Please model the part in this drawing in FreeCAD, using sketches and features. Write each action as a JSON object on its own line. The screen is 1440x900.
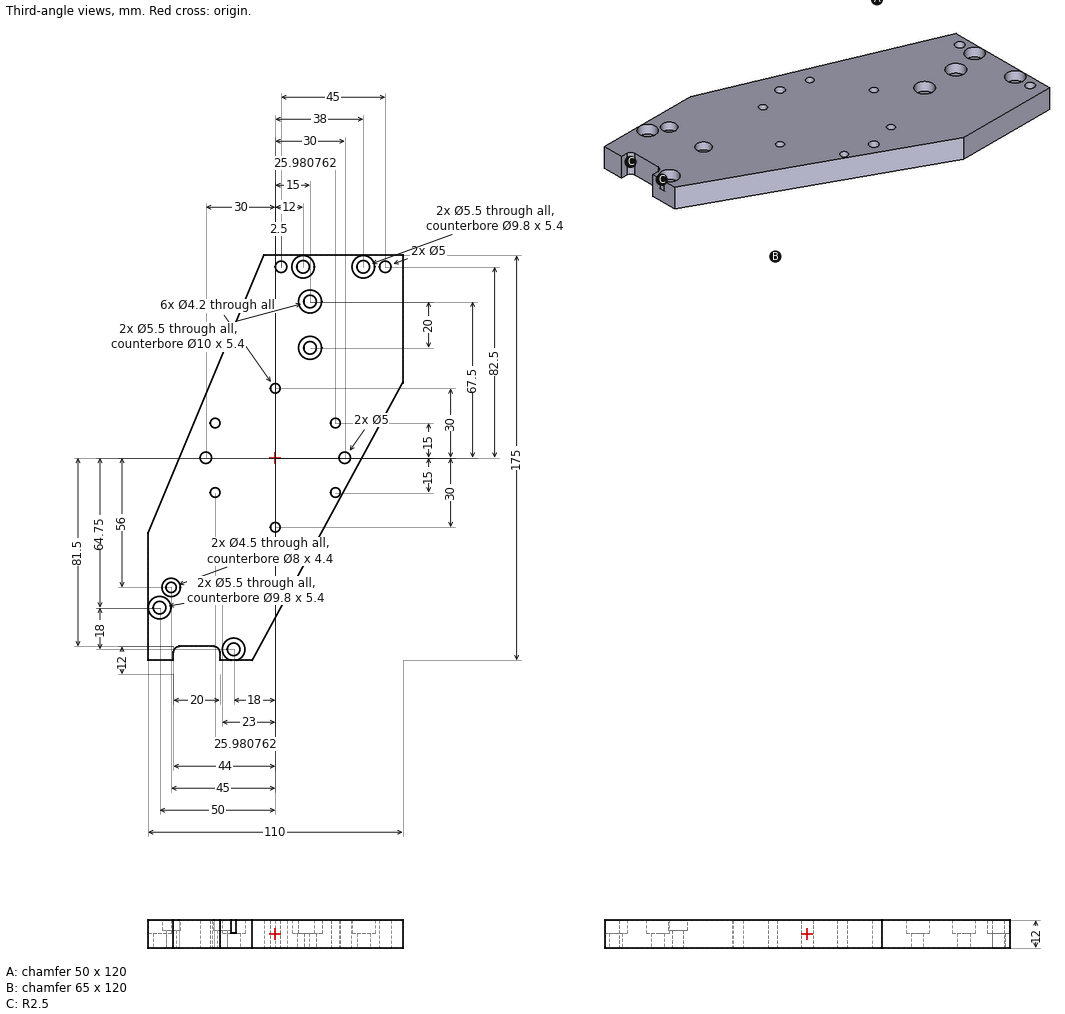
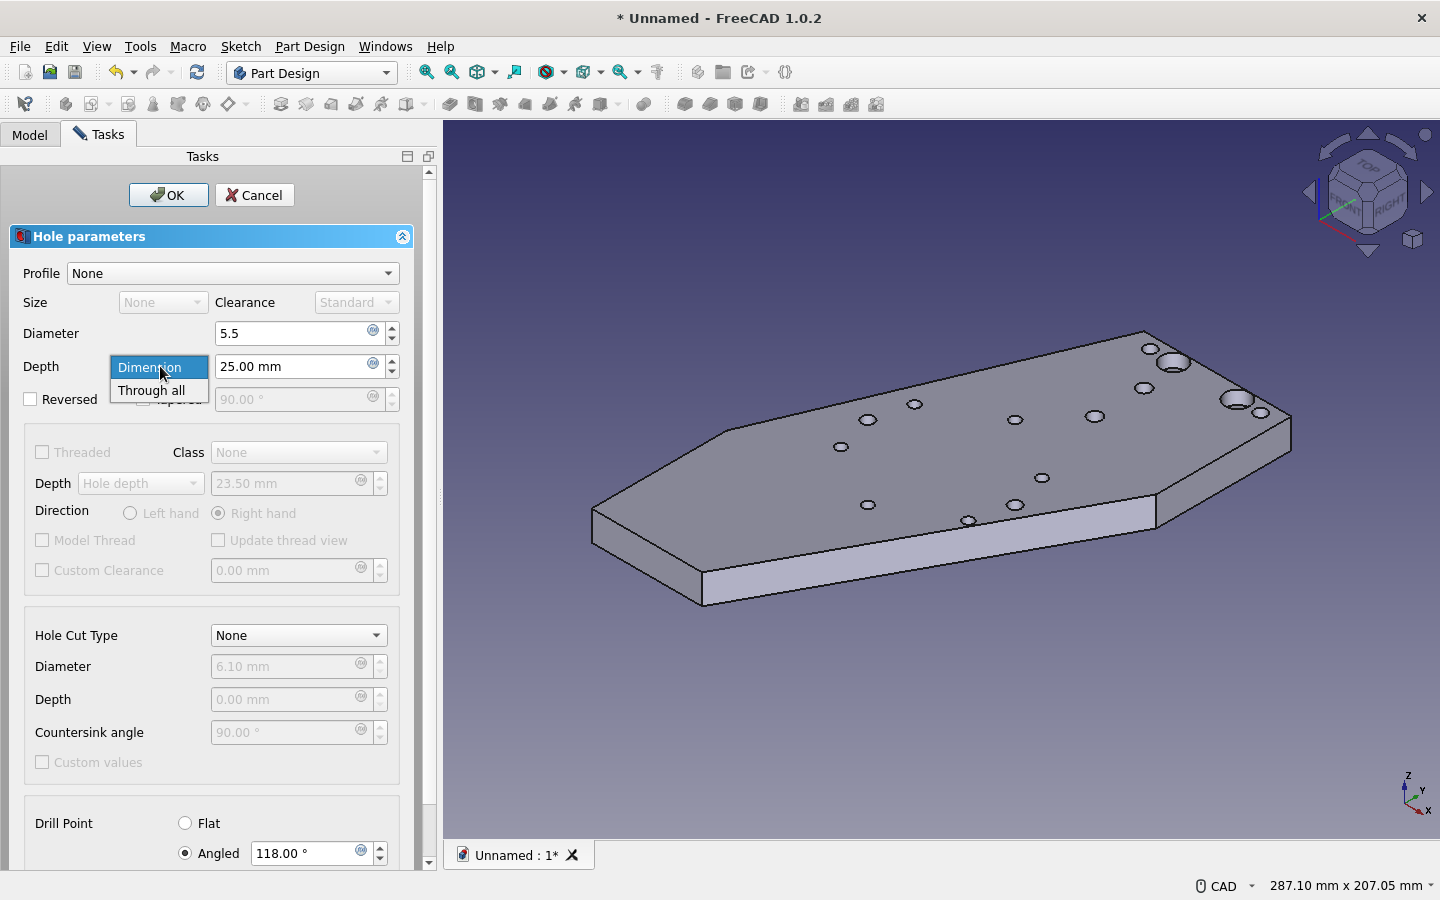
{"action": "left_click", "coordinate": [158, 390]}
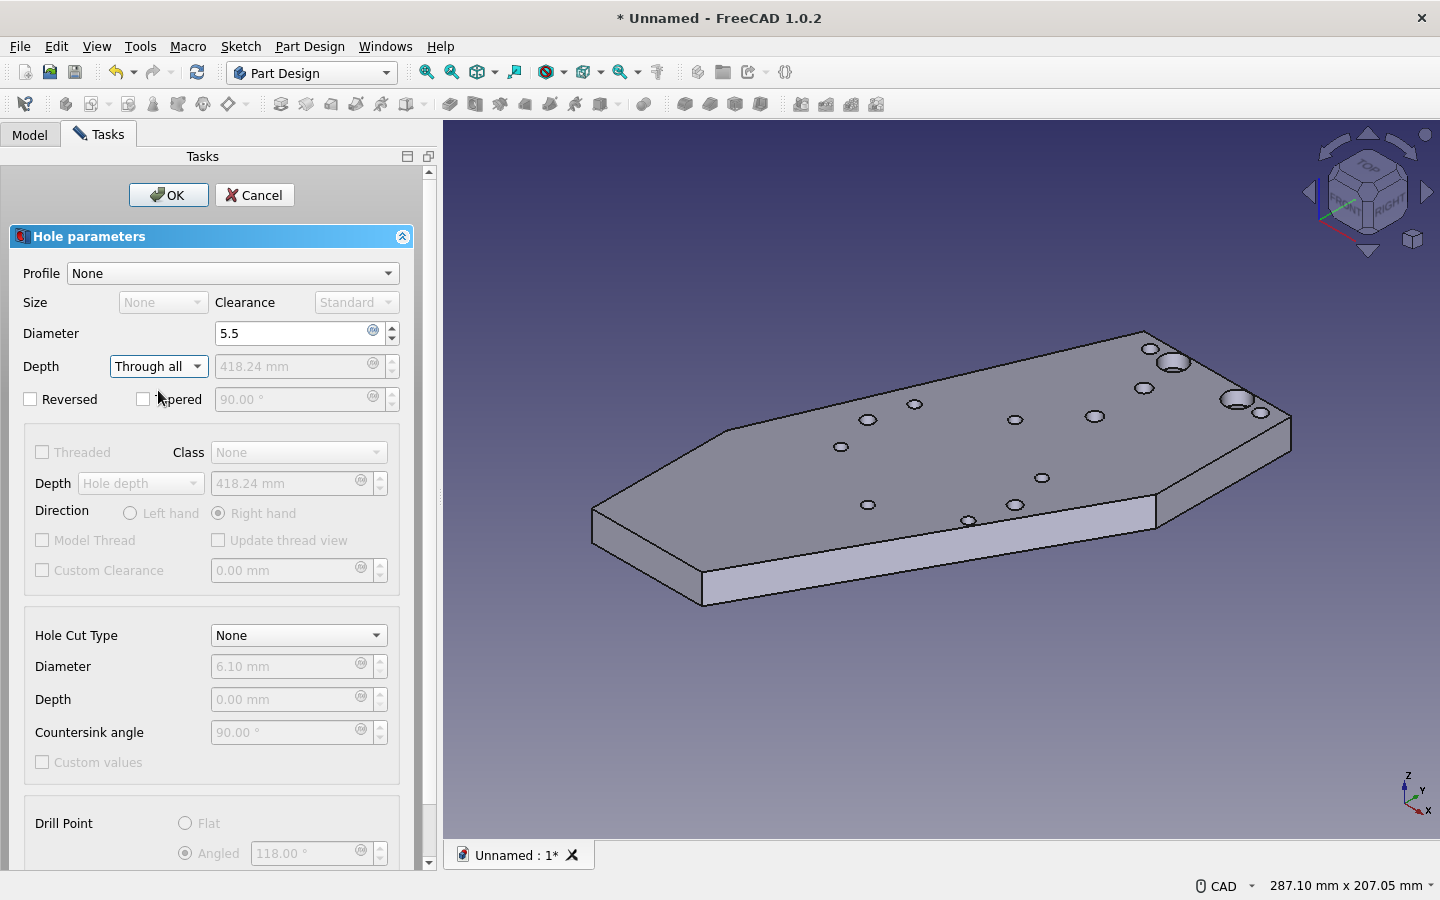
{"action": "left_click", "coordinate": [300, 636]}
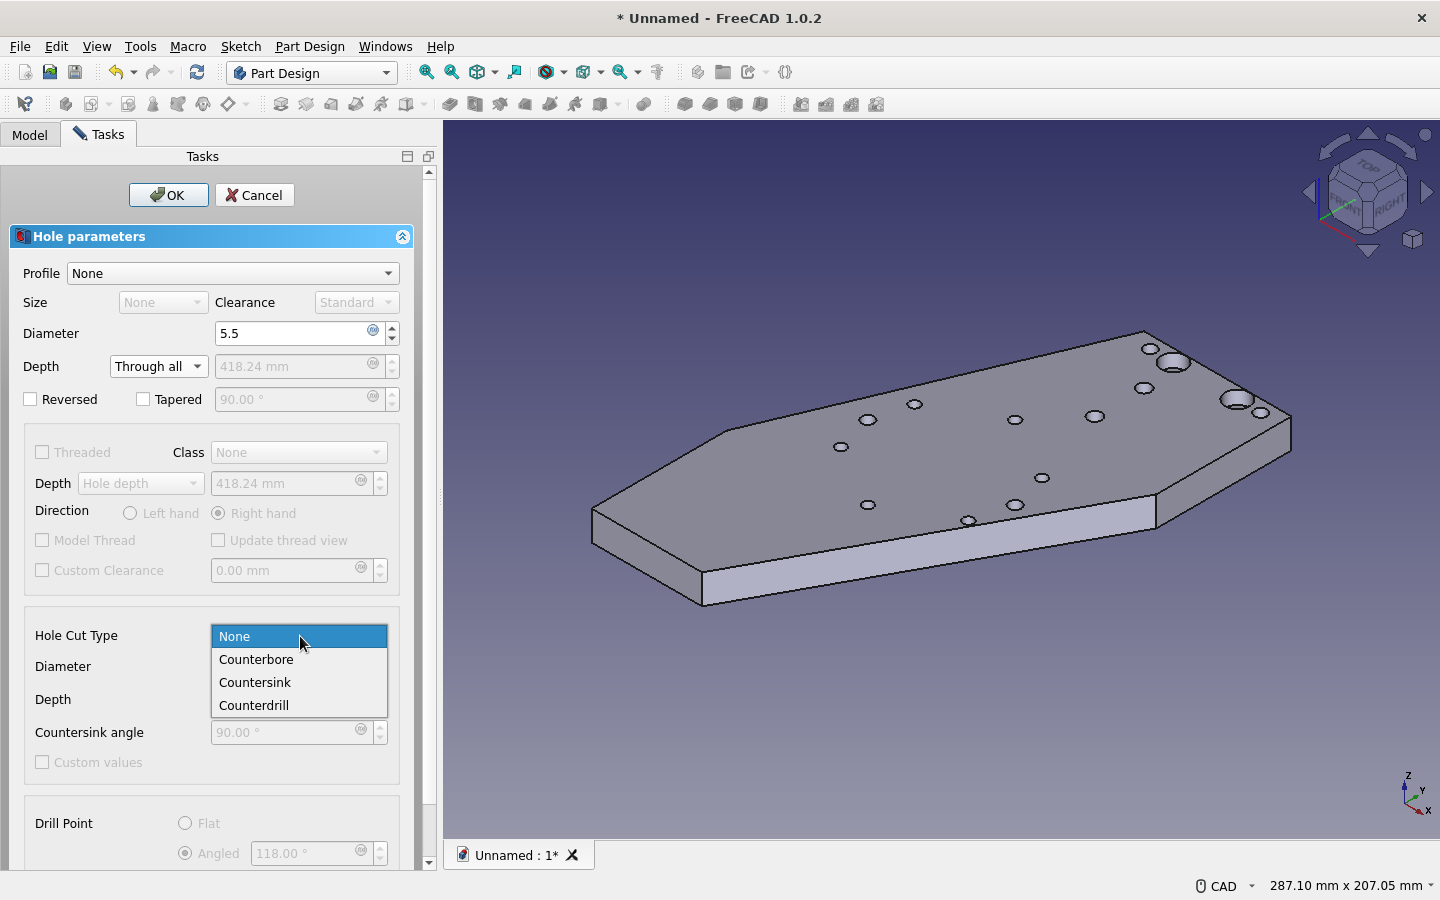
{"action": "left_click", "coordinate": [298, 660]}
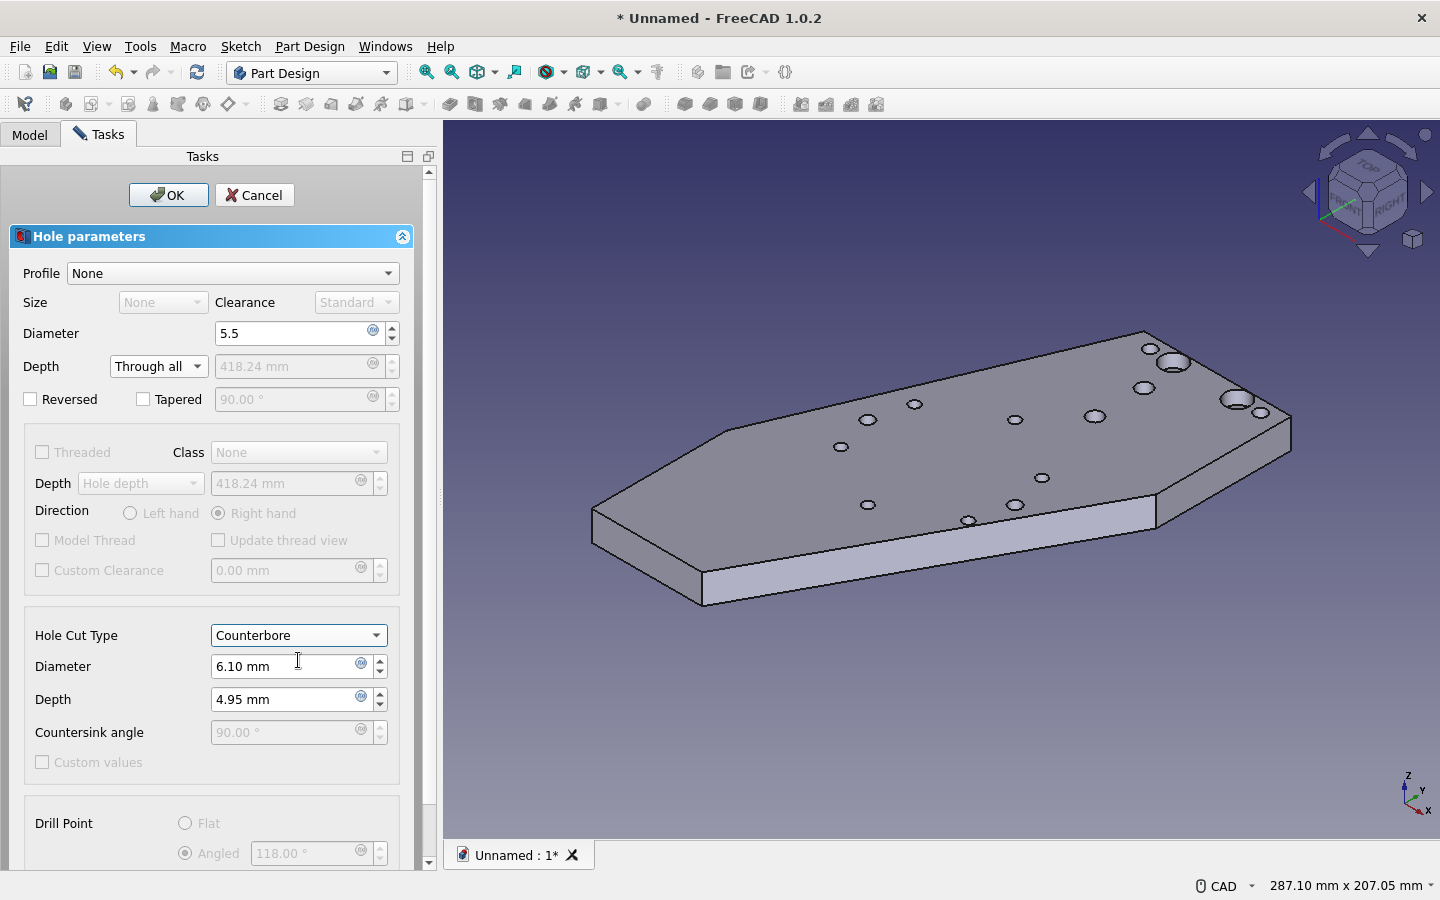
{"action": "triple_click", "coordinate": [292, 666]}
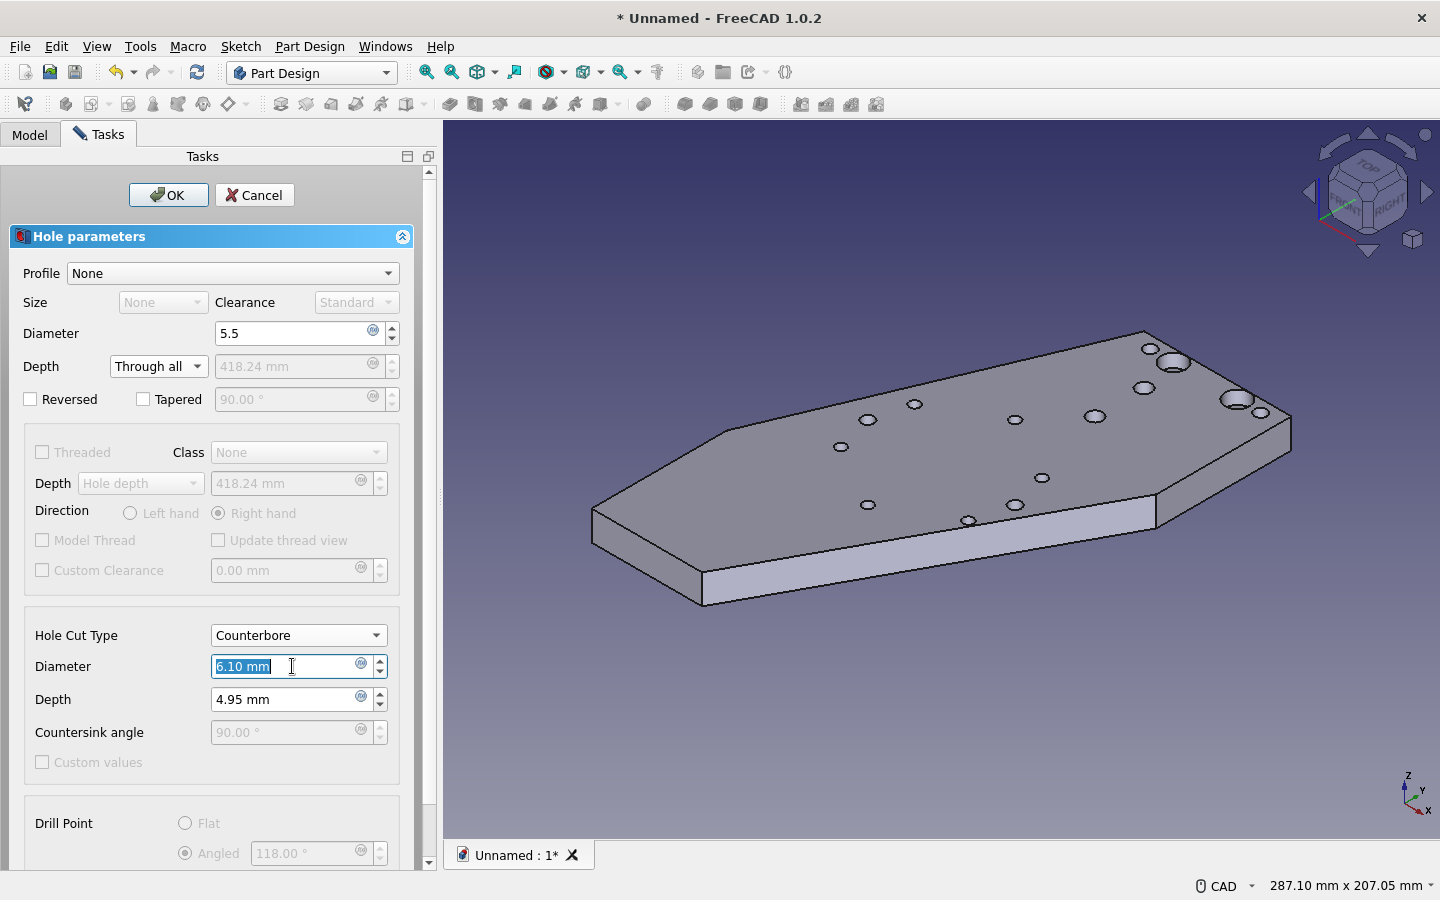
{"action": "type", "text": "10"}
{"action": "key", "text": "Tab"}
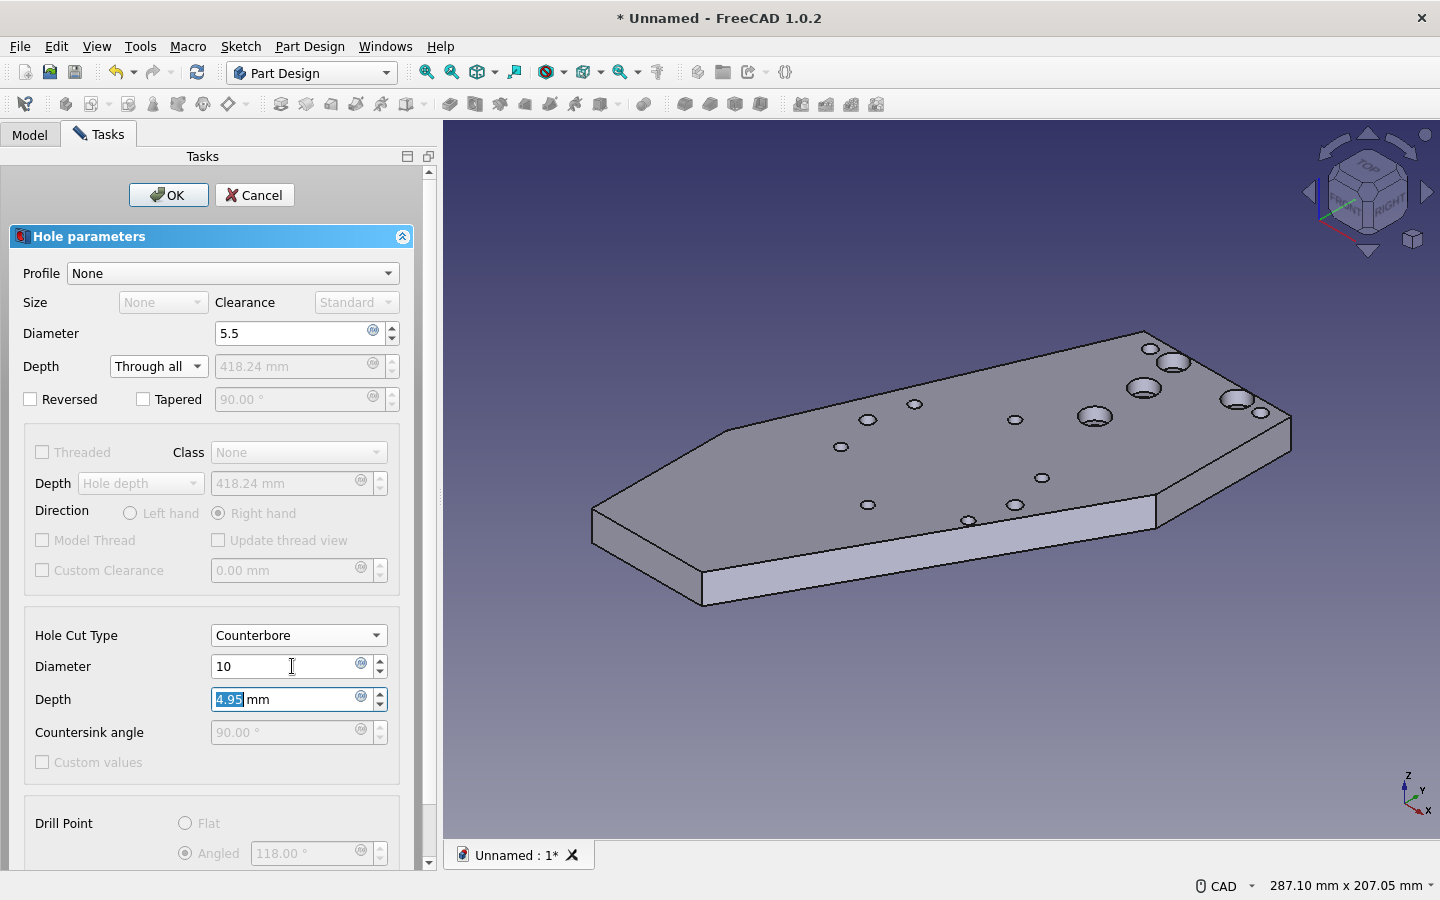
{"action": "type", "text": "5.4"}
{"action": "key", "text": "Tab"}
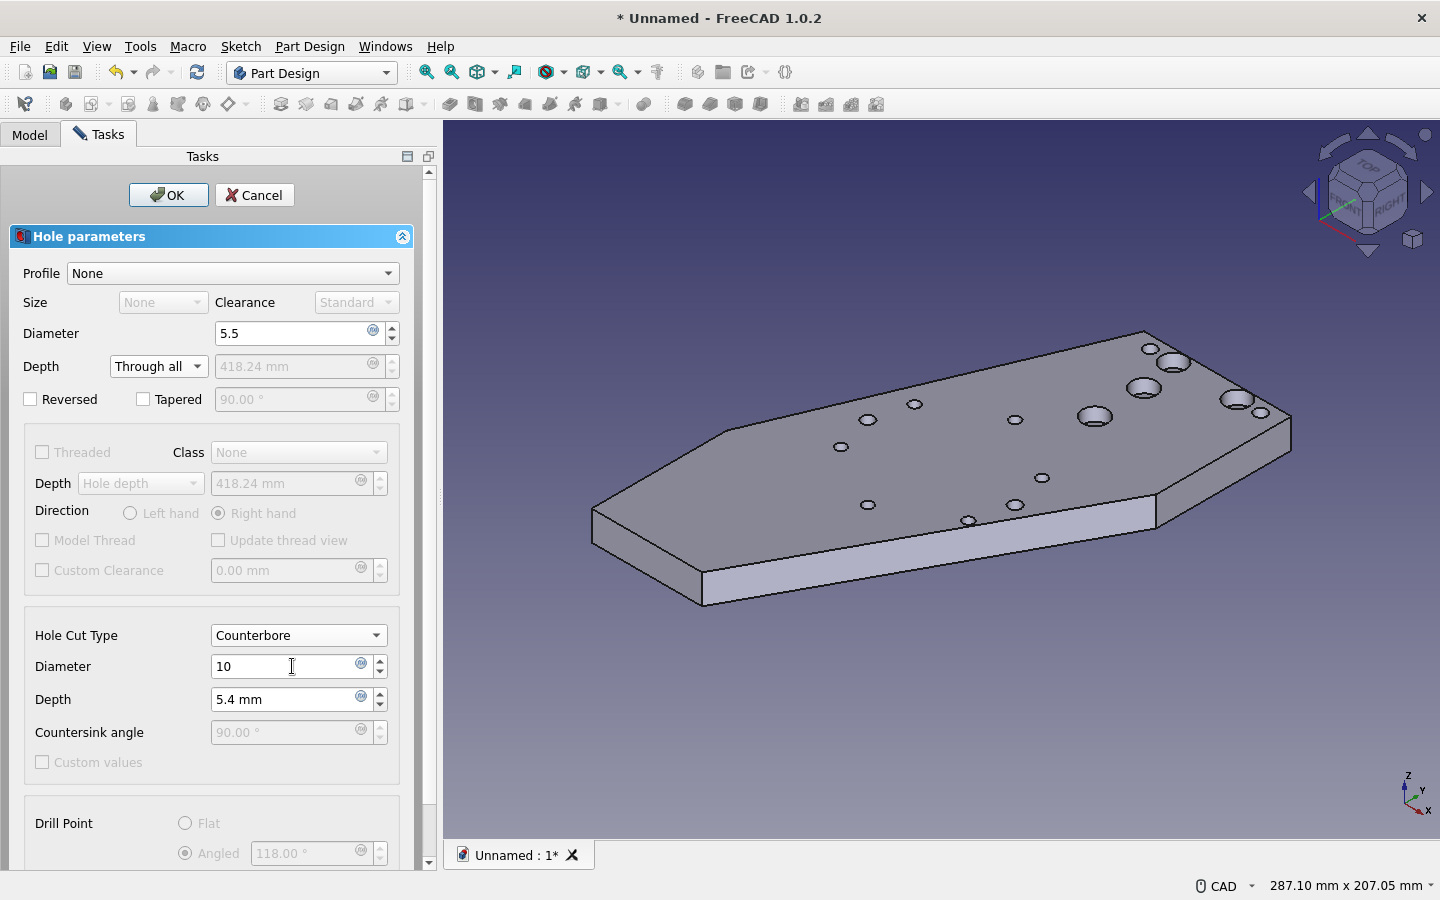
{"action": "left_click", "coordinate": [169, 195]}